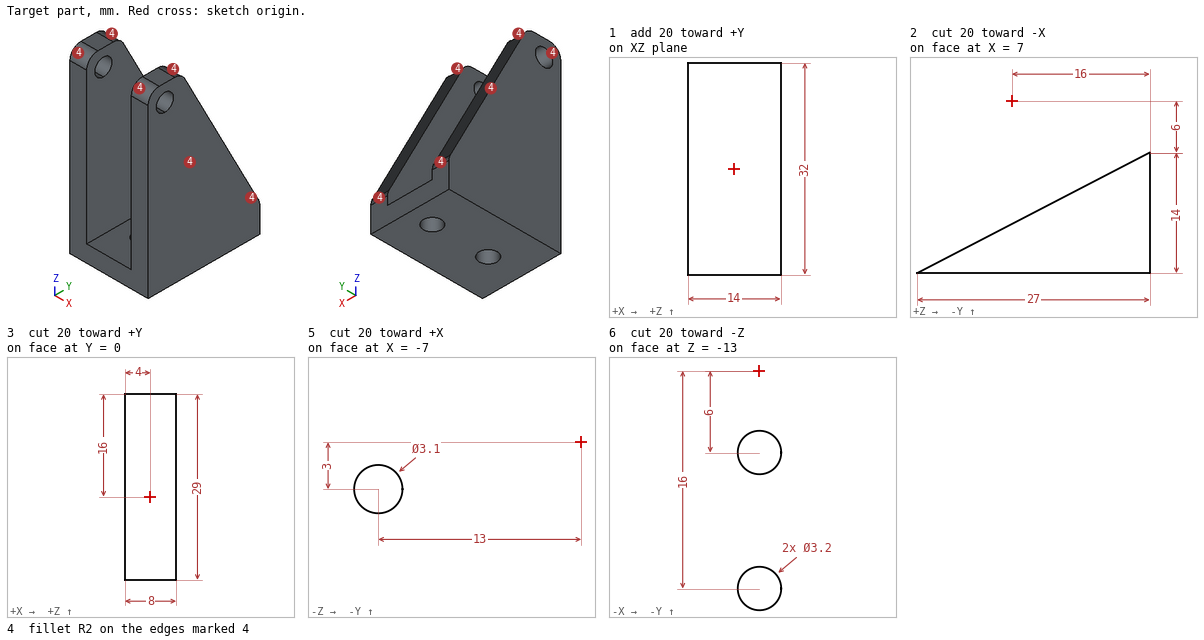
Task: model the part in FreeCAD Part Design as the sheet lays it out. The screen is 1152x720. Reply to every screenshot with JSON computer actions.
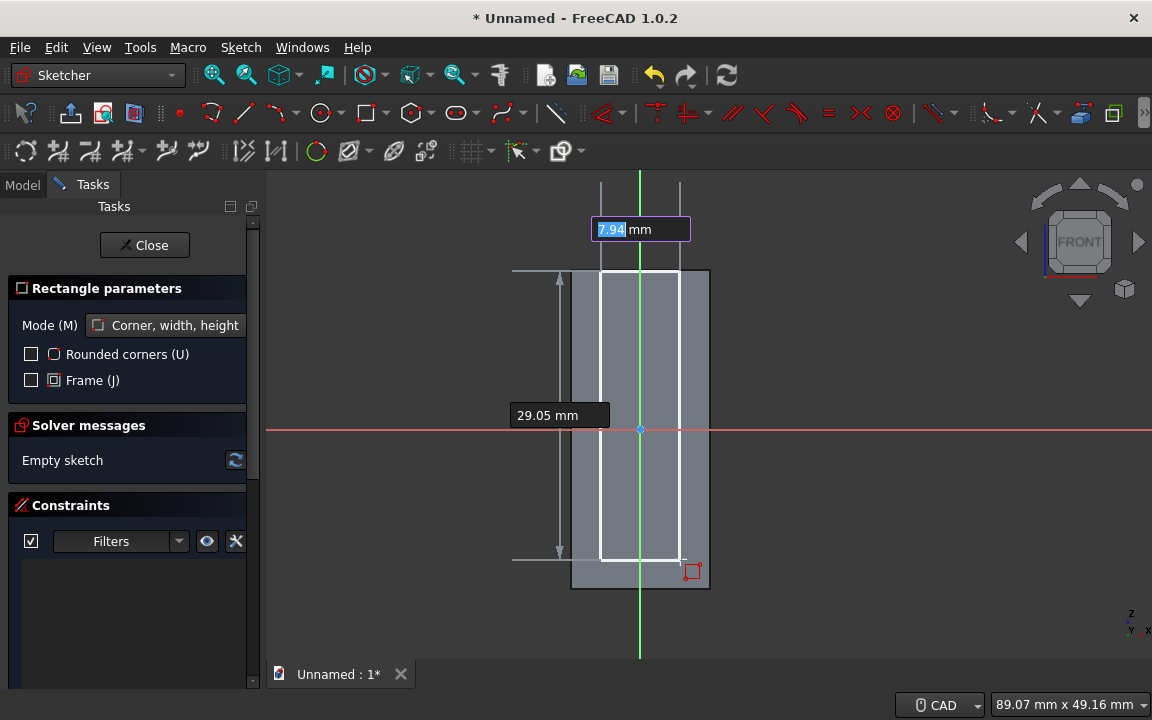
{"action": "type", "text": "8"}
{"action": "key", "text": "Tab"}
{"action": "type", "text": "29"}
{"action": "key", "text": "Return"}
{"action": "key", "text": "Escape"}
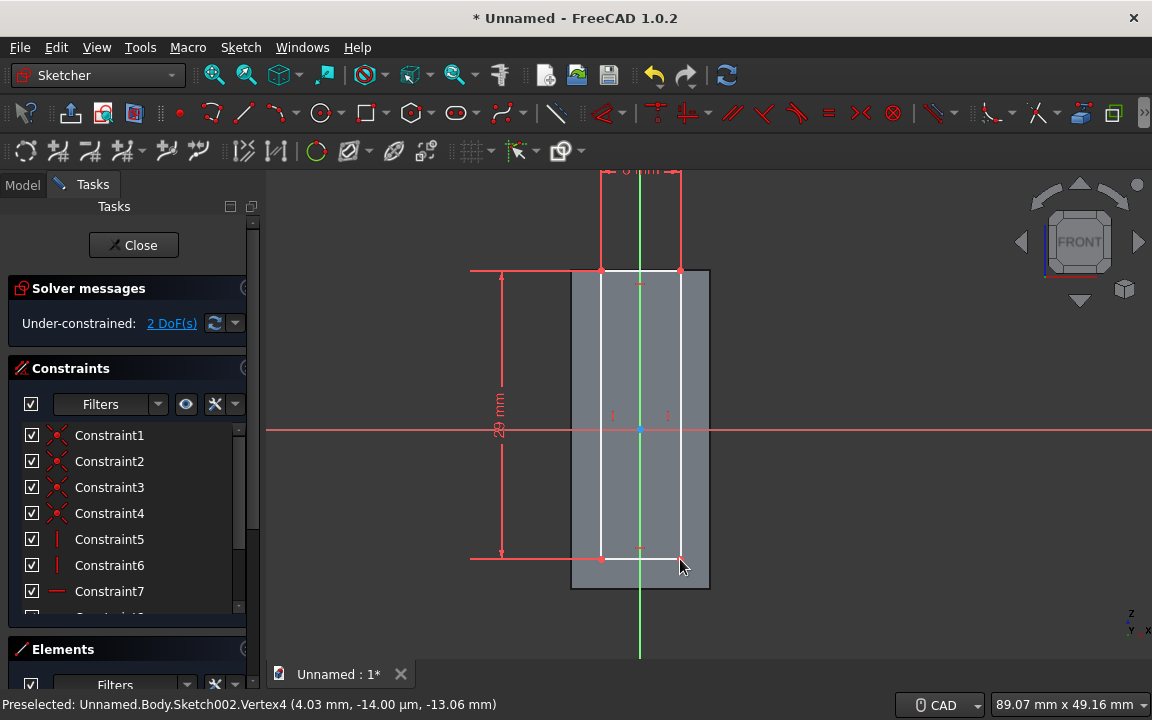
{"action": "left_click", "coordinate": [602, 114]}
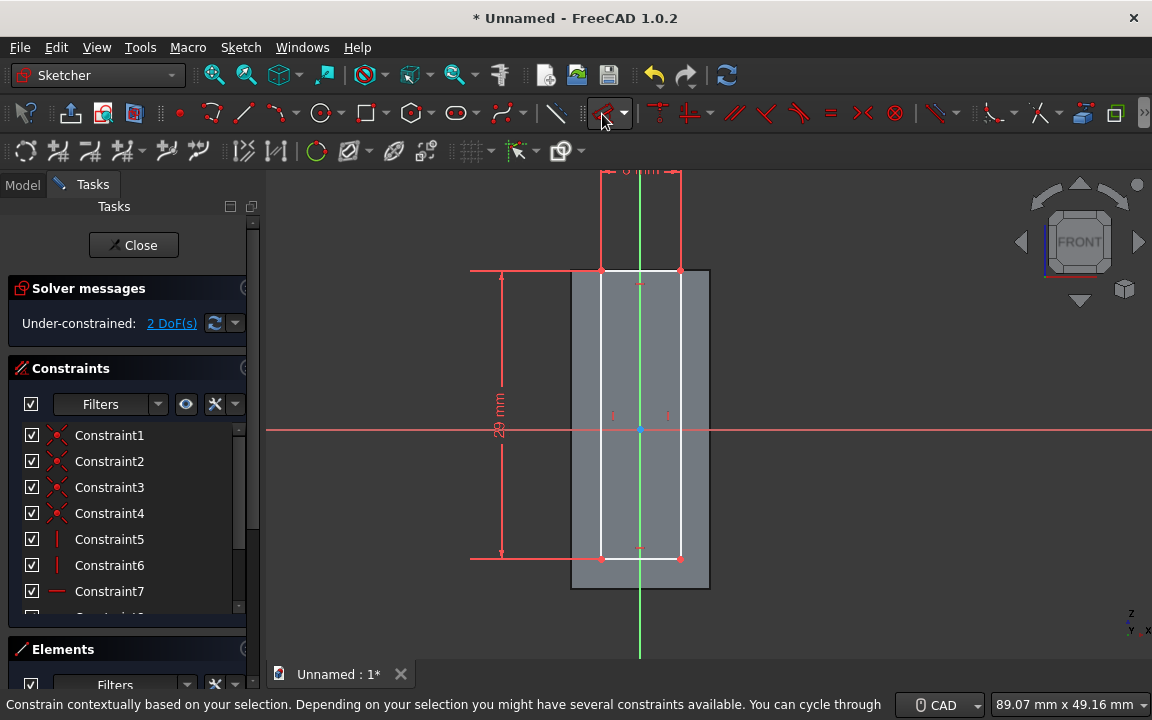
{"action": "left_click", "coordinate": [601, 271]}
{"action": "left_click", "coordinate": [621, 237]}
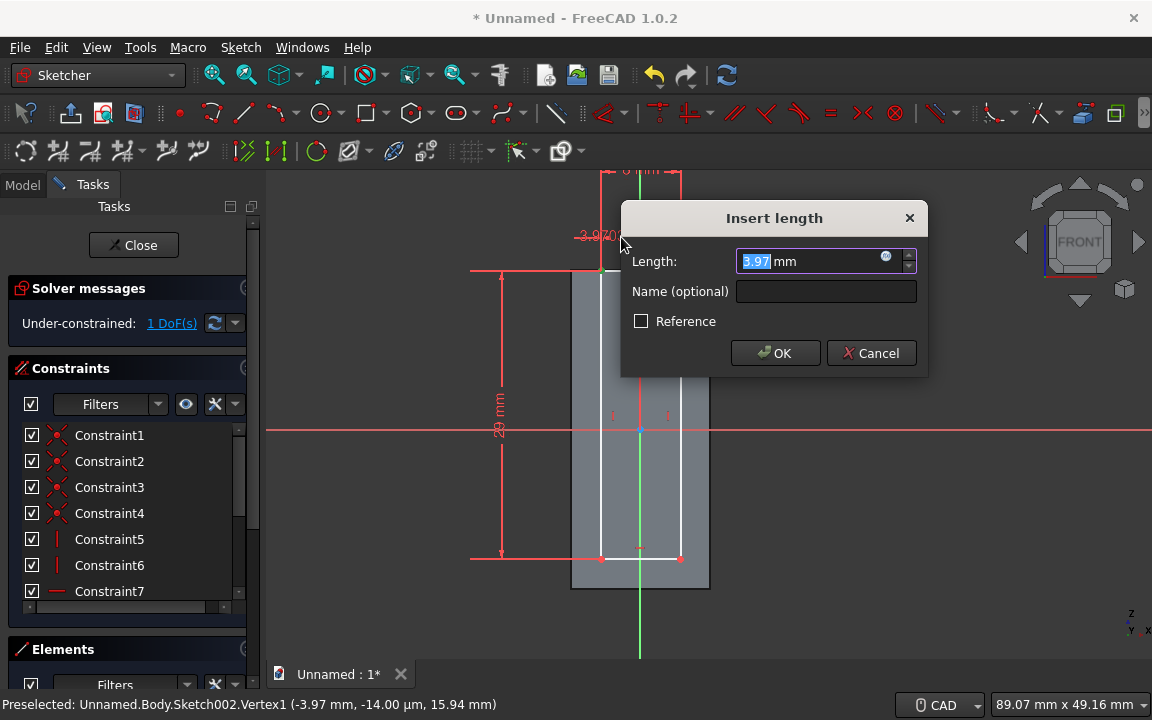
{"action": "type", "text": "4"}
{"action": "key", "text": "Return"}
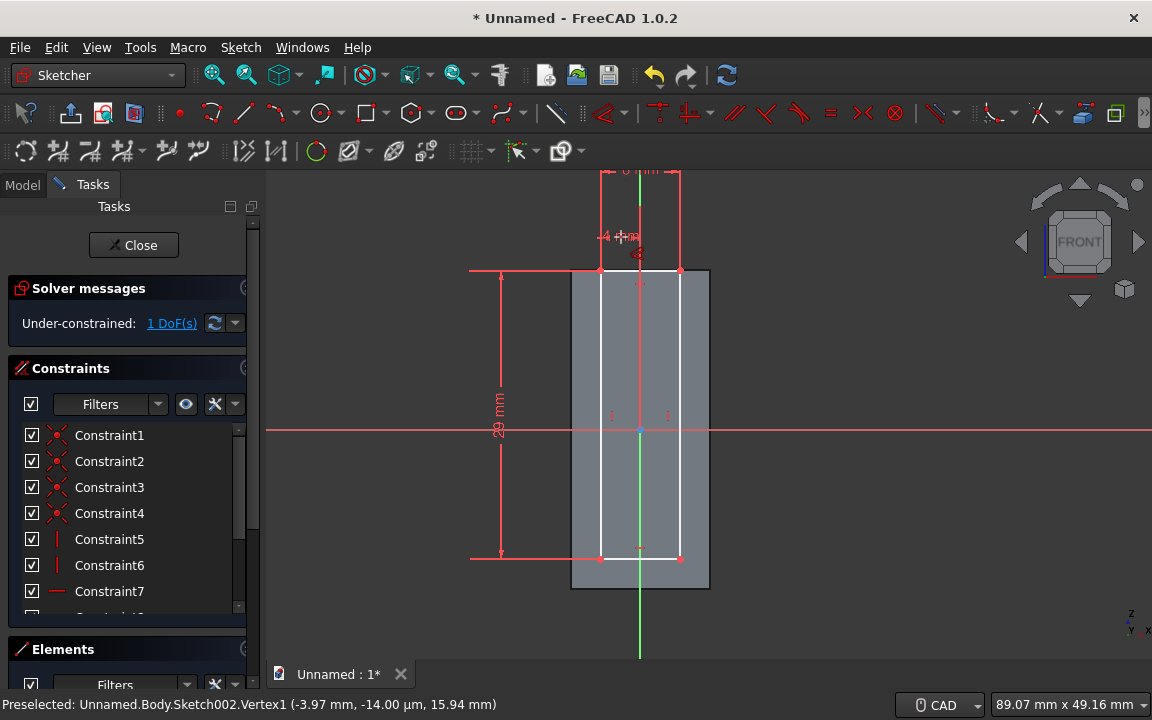
{"action": "left_click", "coordinate": [601, 271]}
{"action": "left_click", "coordinate": [567, 350]}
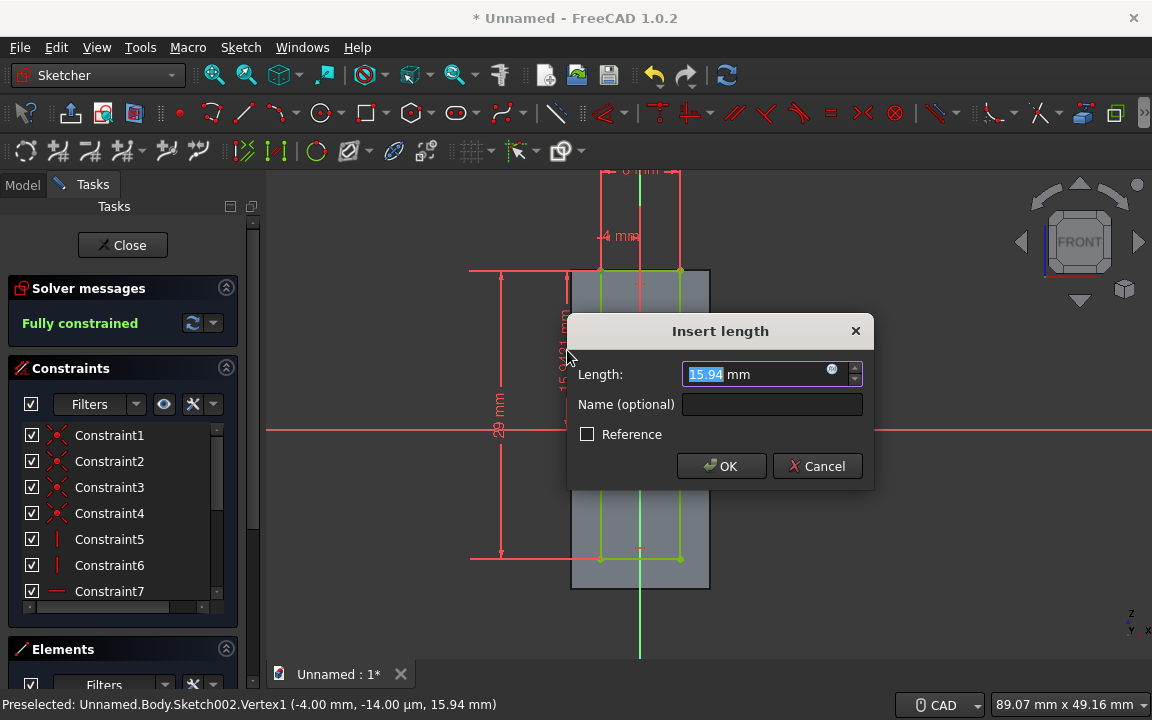
{"action": "type", "text": "16"}
{"action": "key", "text": "Return"}
{"action": "key", "text": "Escape"}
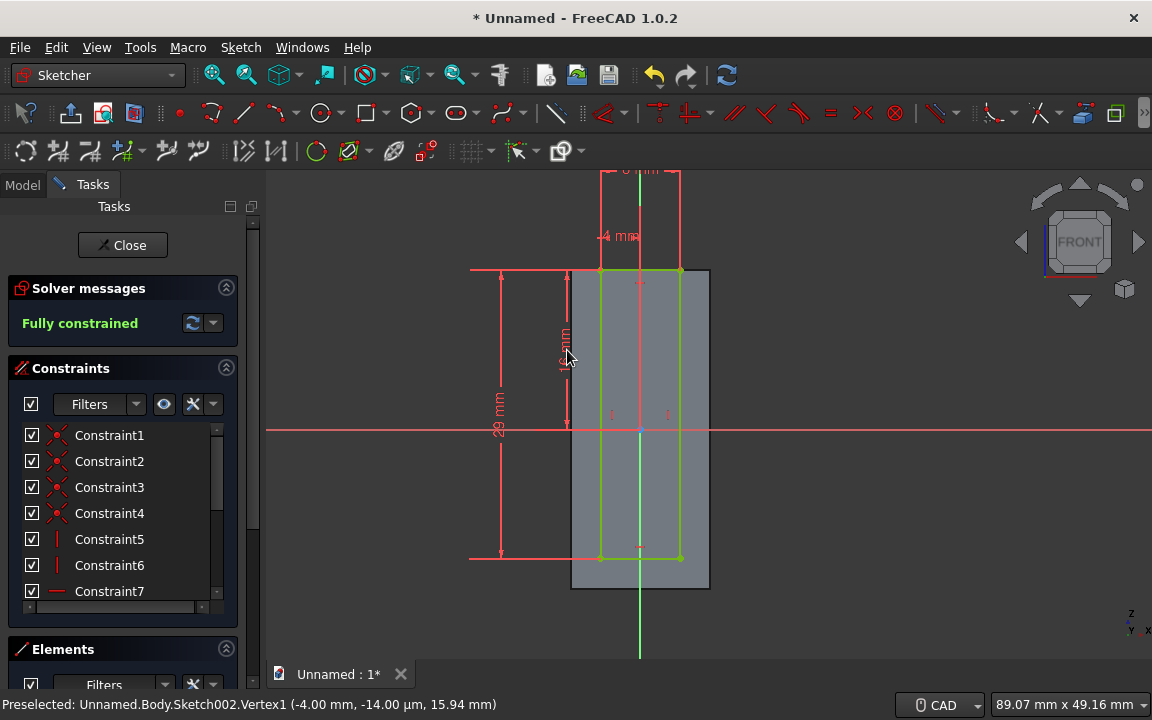
{"action": "left_click", "coordinate": [123, 245]}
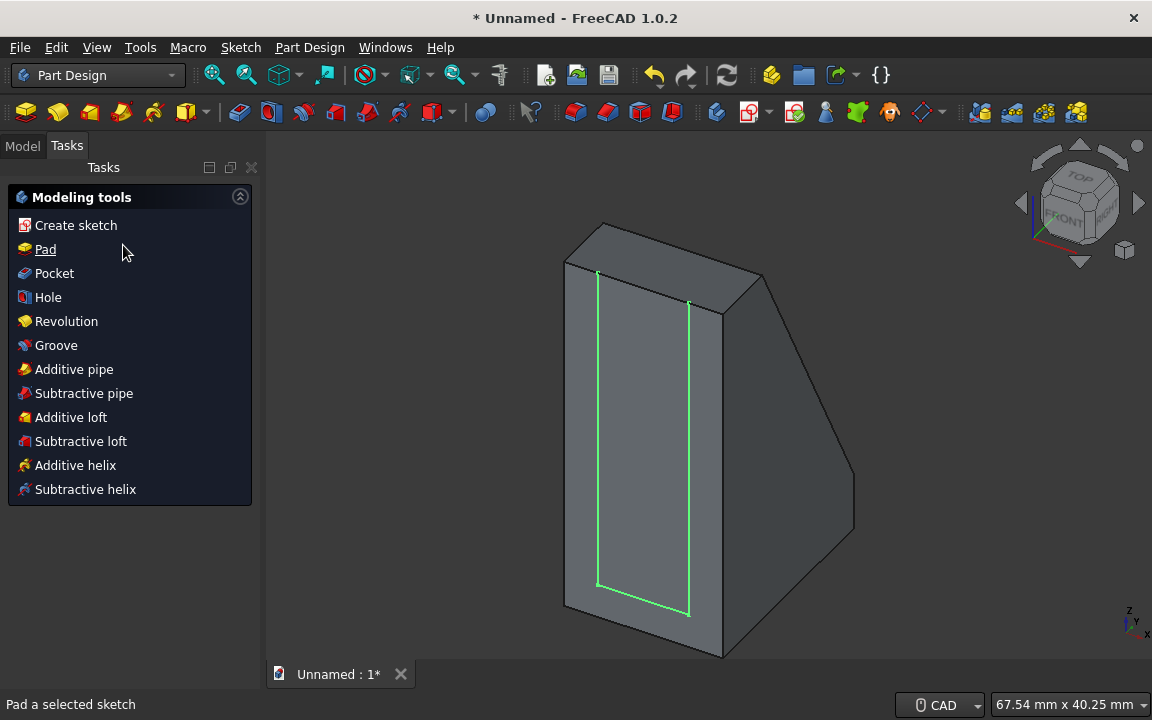
{"action": "left_click", "coordinate": [240, 112]}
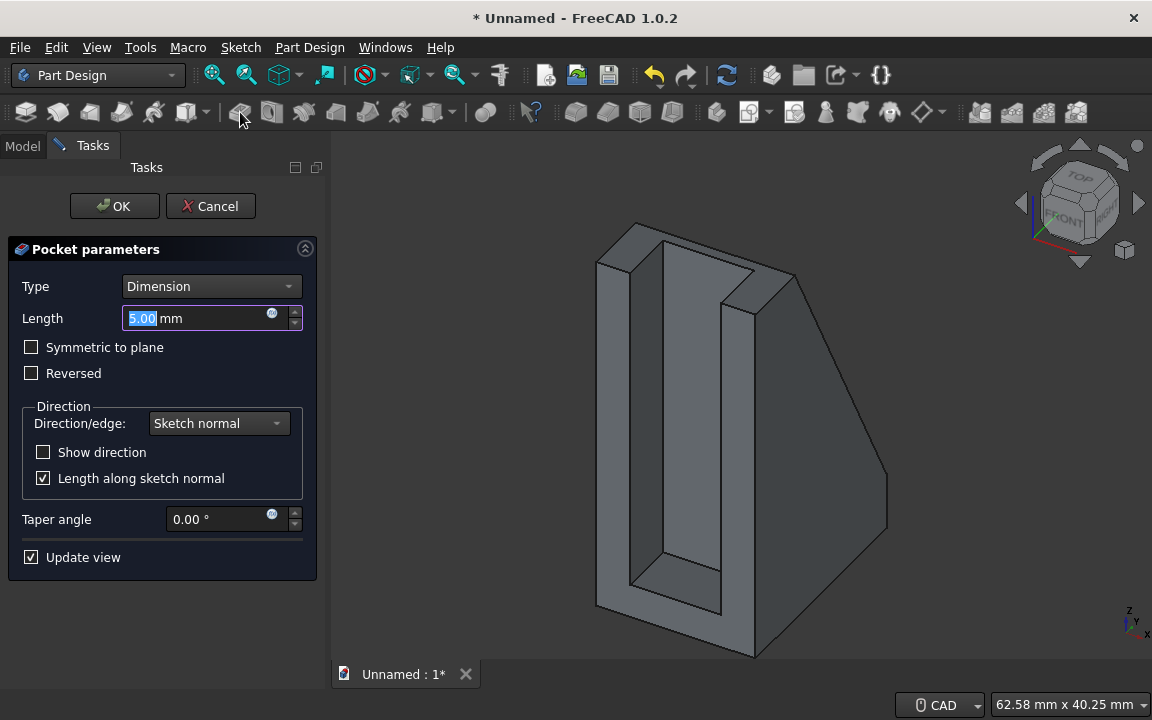
{"action": "type", "text": "20"}
{"action": "key", "text": "Tab"}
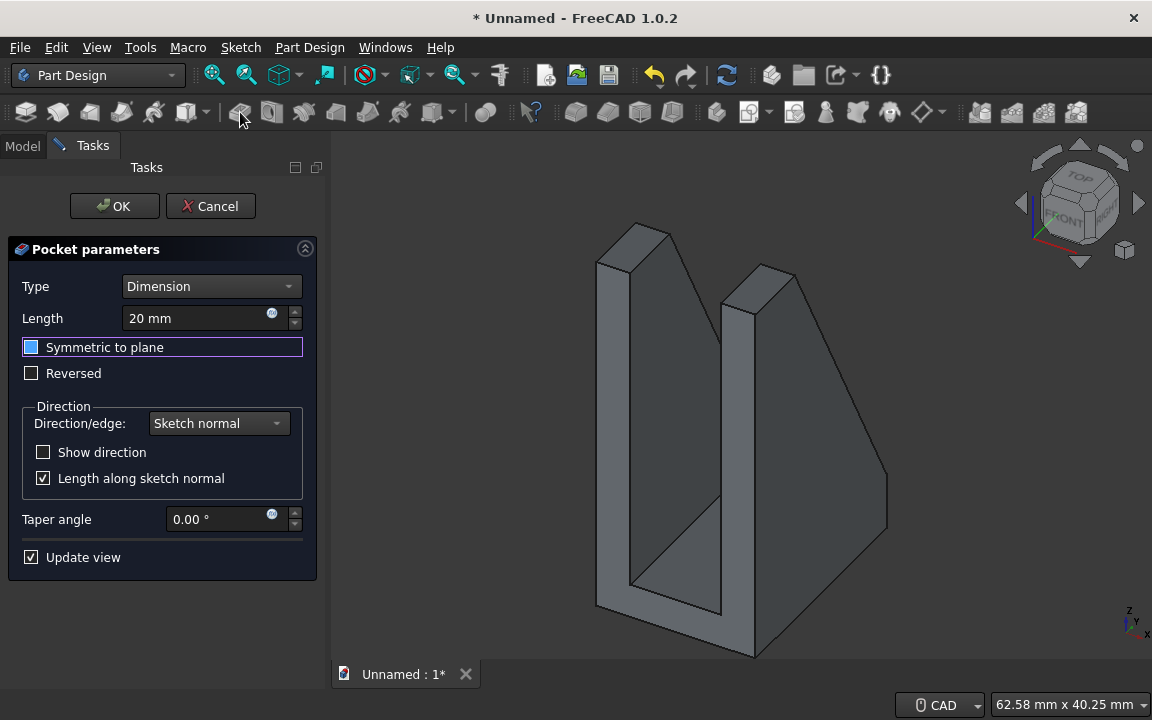
{"action": "left_click", "coordinate": [115, 206]}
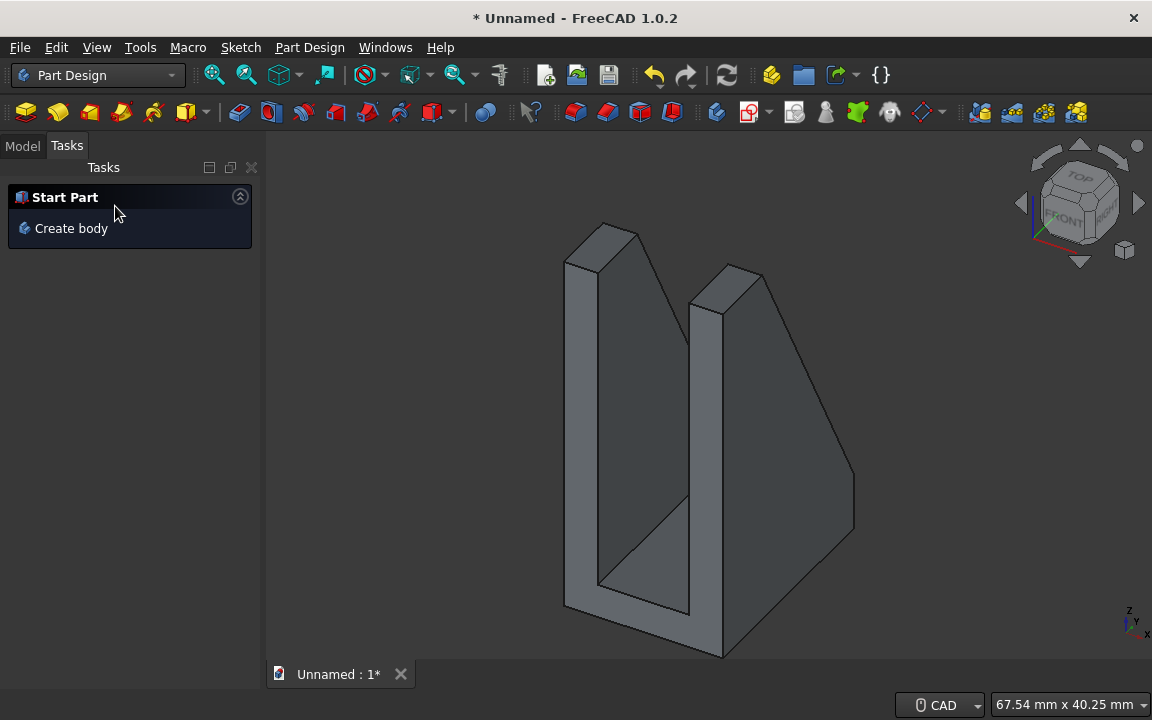
{"action": "left_click", "coordinate": [706, 308]}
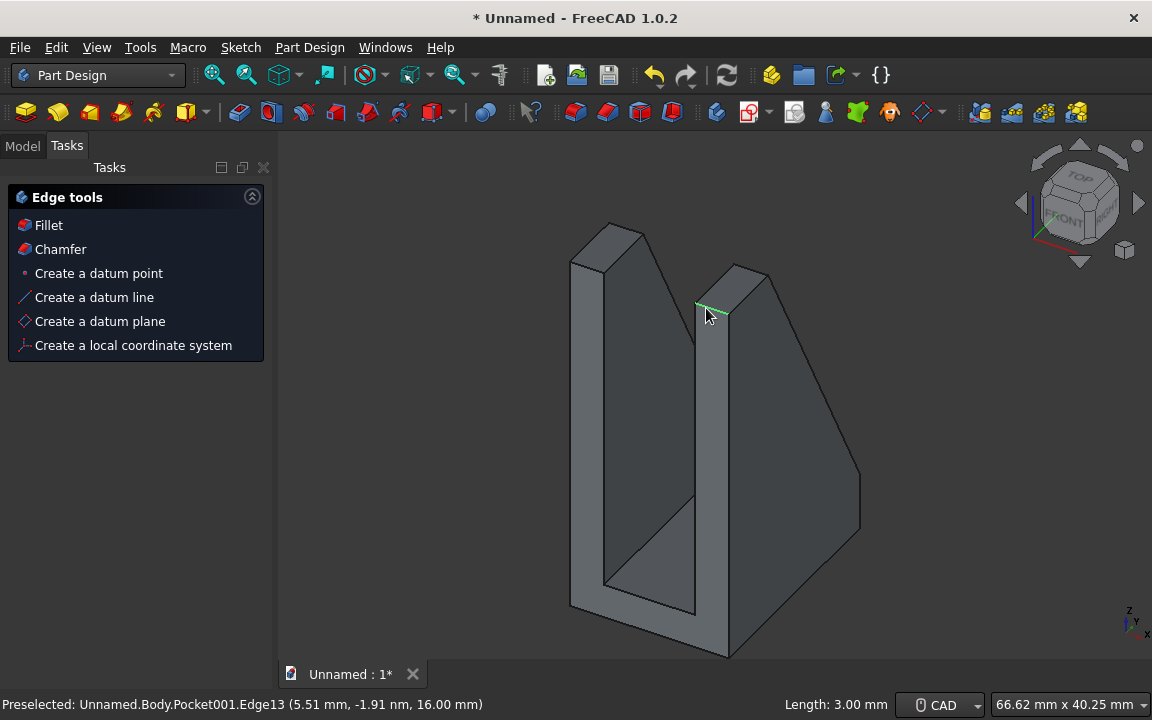
{"action": "left_click", "coordinate": [587, 267], "text": "ctrl"}